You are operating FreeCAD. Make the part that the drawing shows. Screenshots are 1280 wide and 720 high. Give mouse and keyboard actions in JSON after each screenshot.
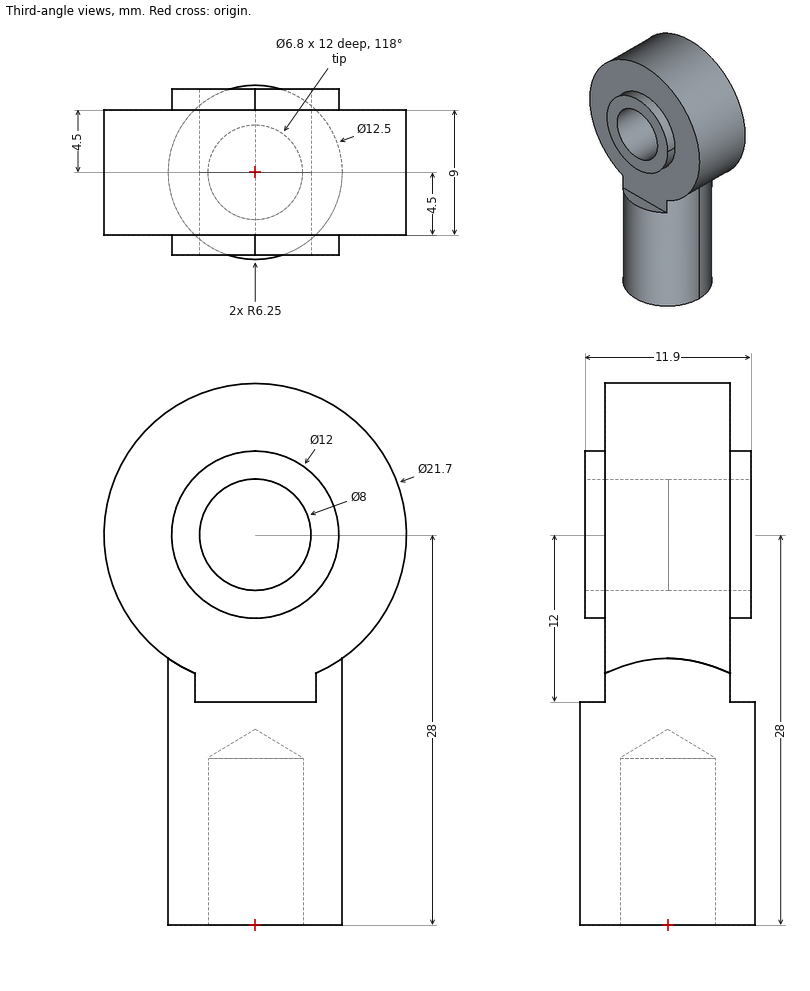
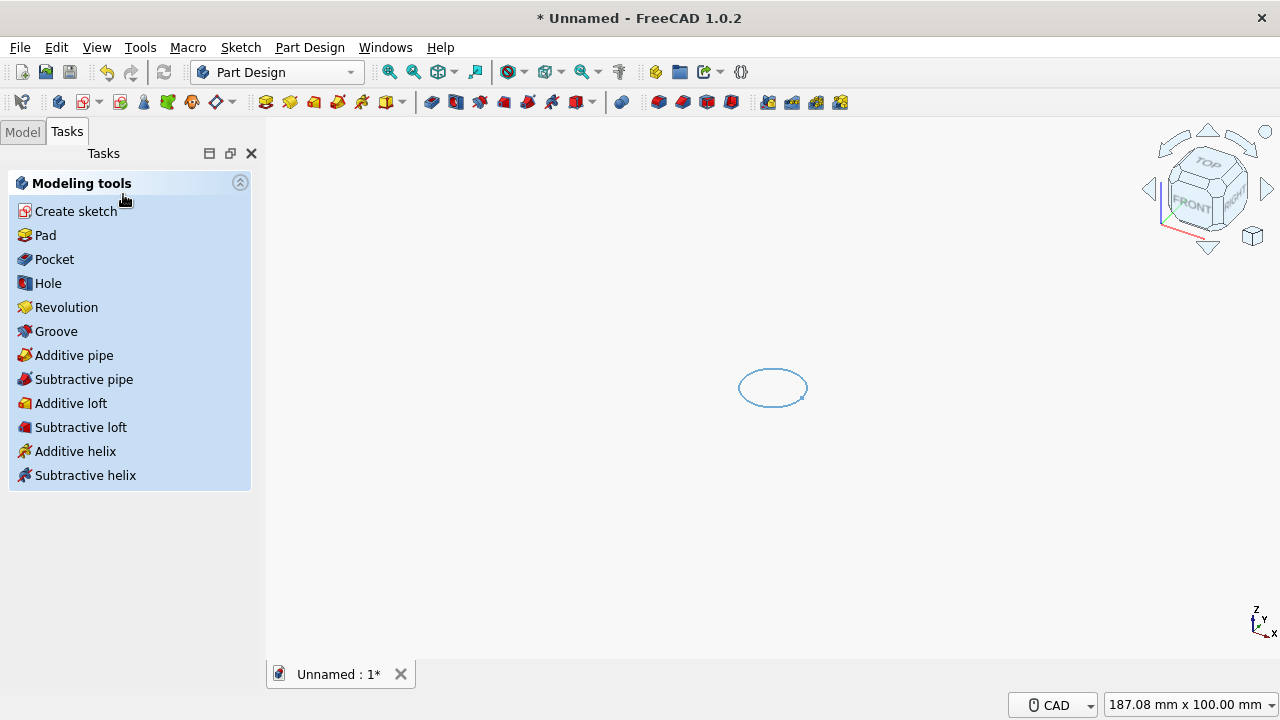
{"action": "left_click", "coordinate": [266, 102]}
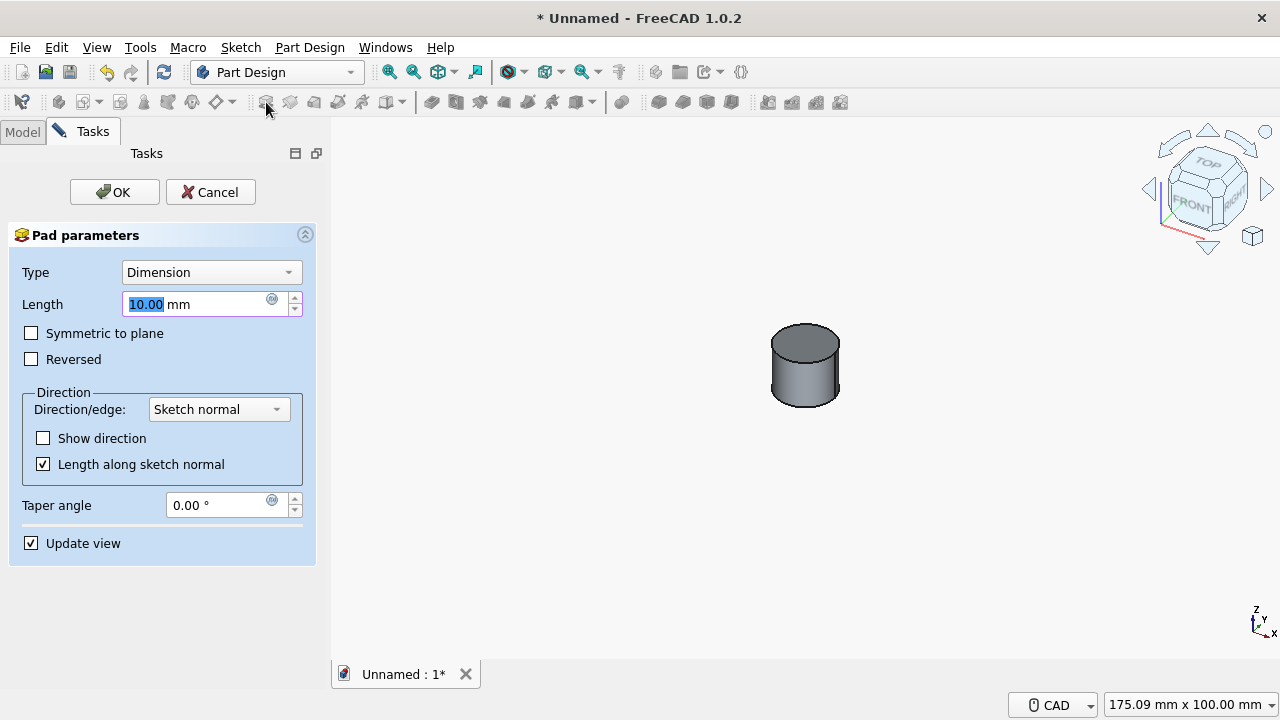
{"action": "type", "text": "28"}
{"action": "key", "text": "Tab"}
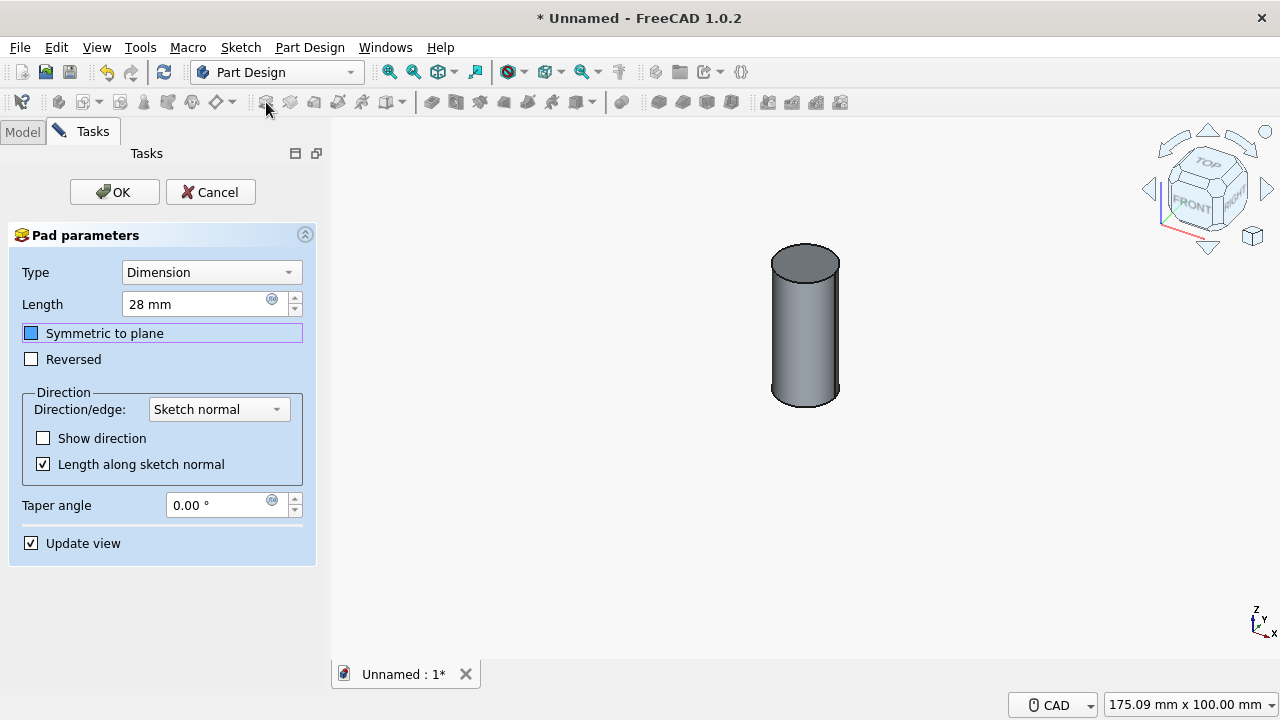
{"action": "left_click", "coordinate": [115, 192]}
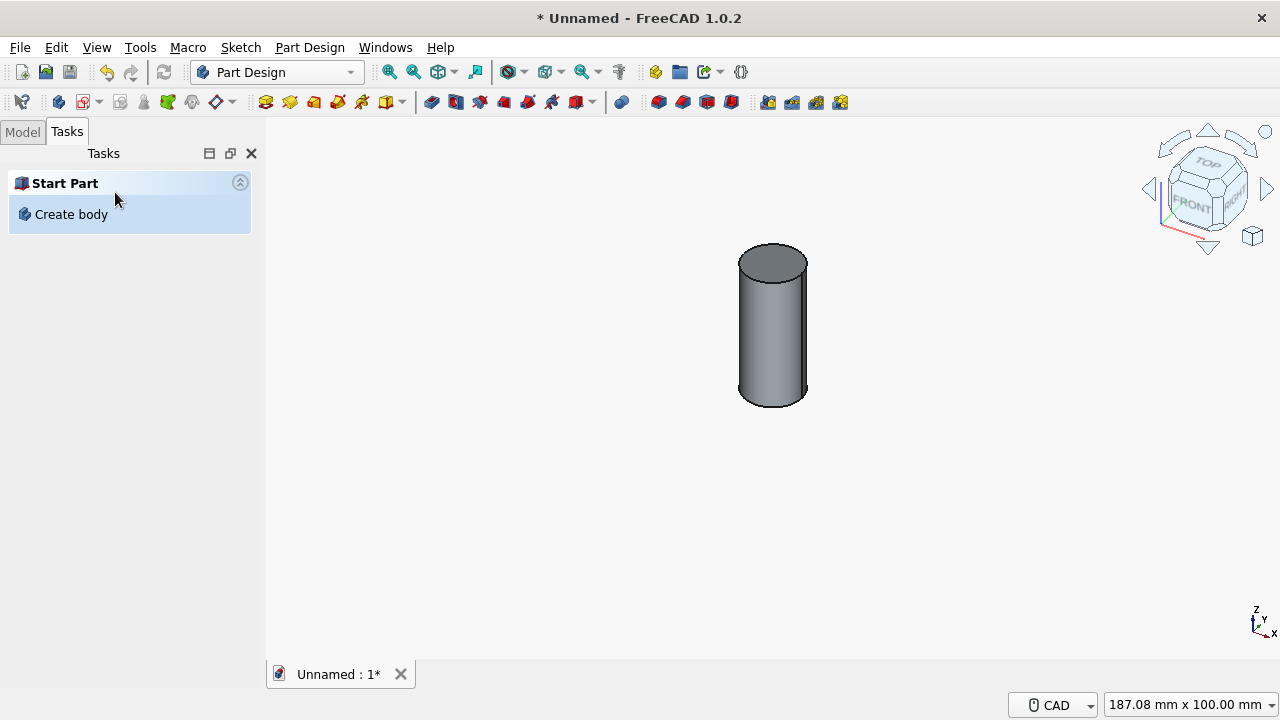
{"action": "left_click", "coordinate": [390, 72]}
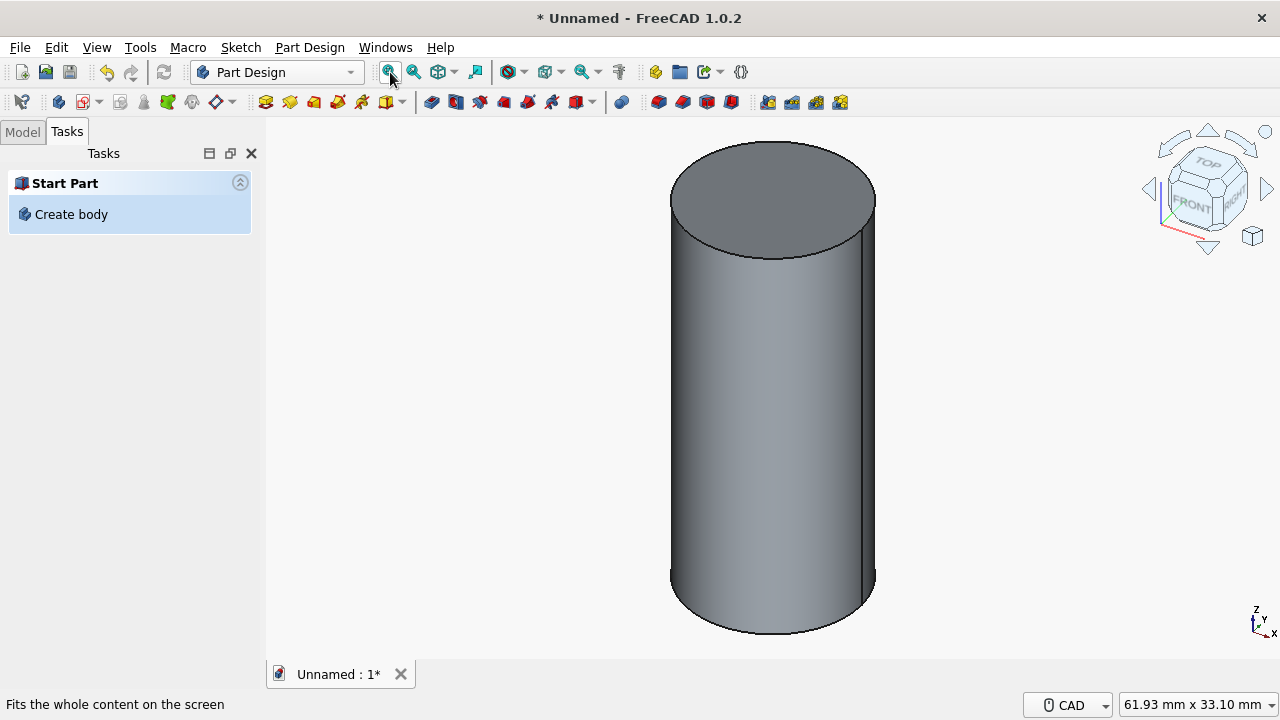
{"action": "left_click", "coordinate": [84, 102]}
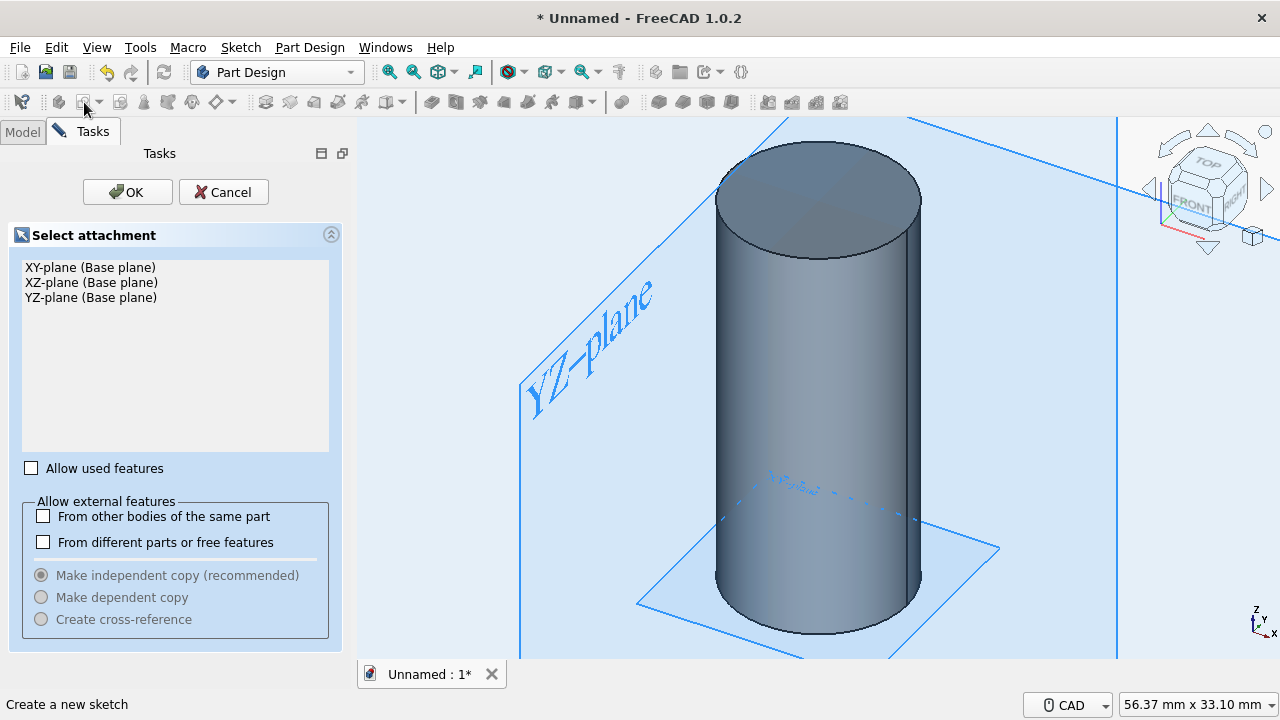
{"action": "left_click", "coordinate": [82, 282]}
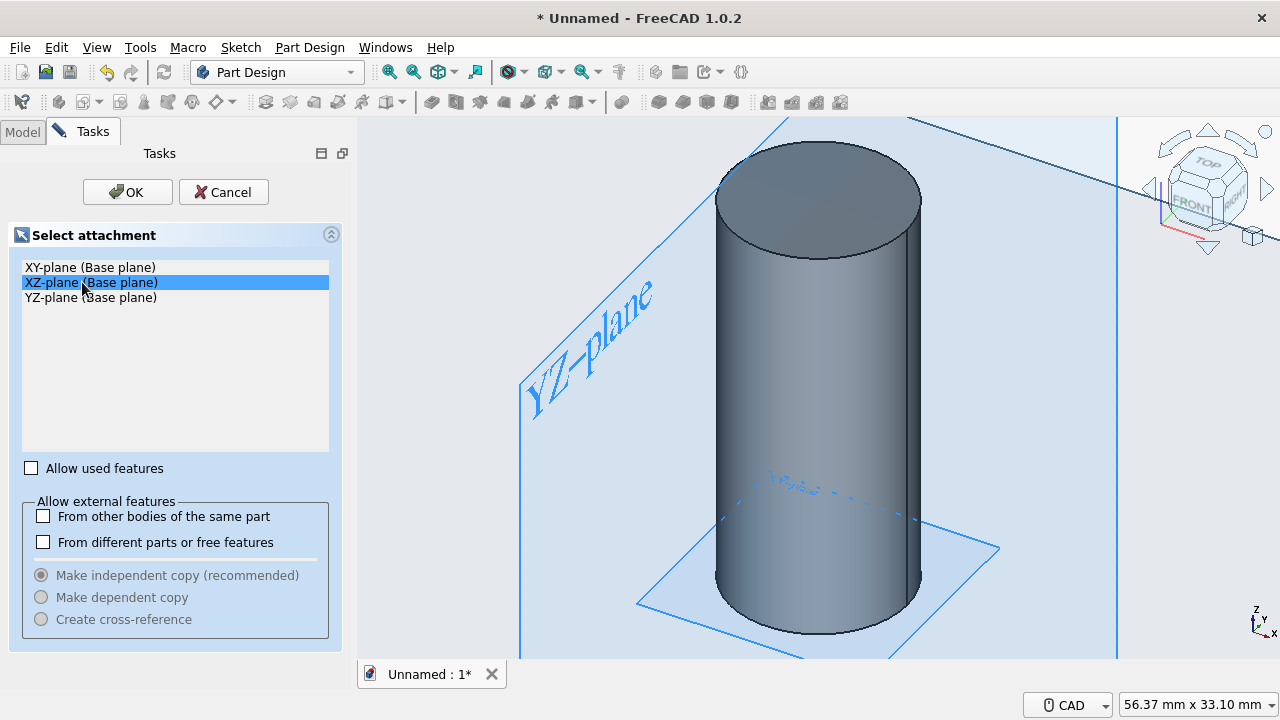
{"action": "left_click", "coordinate": [128, 192]}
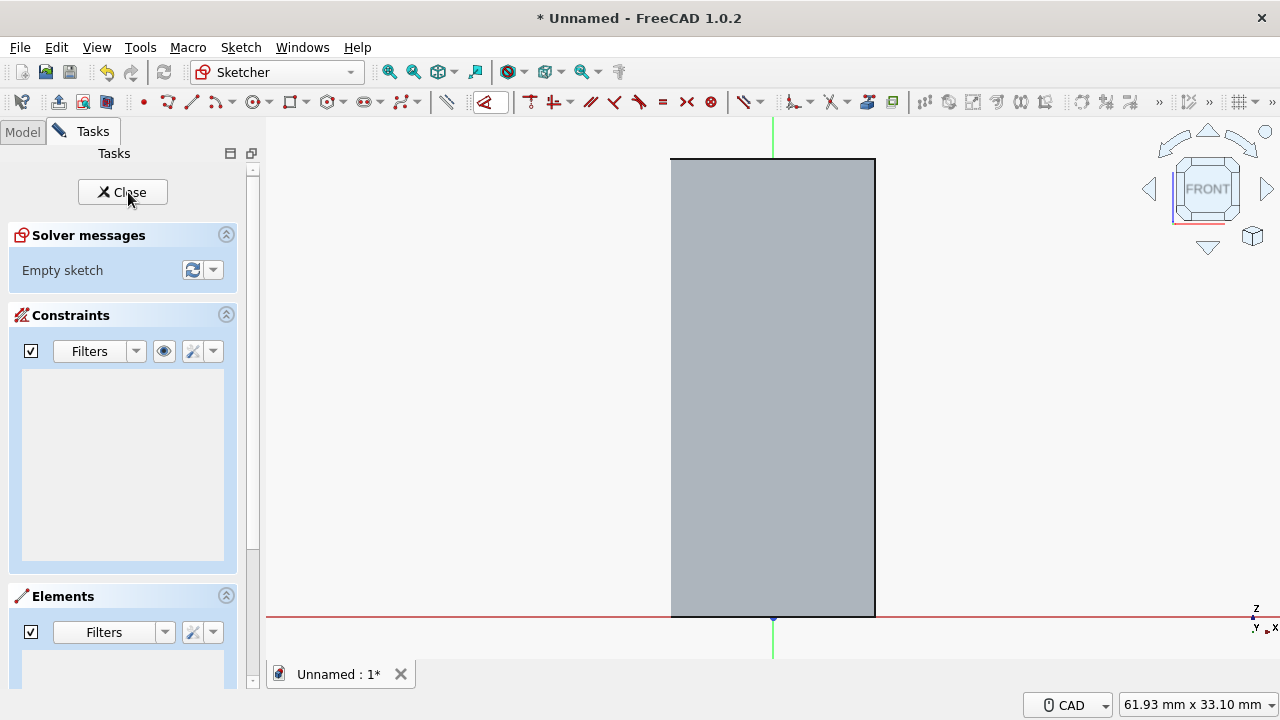
{"action": "left_click", "coordinate": [108, 102]}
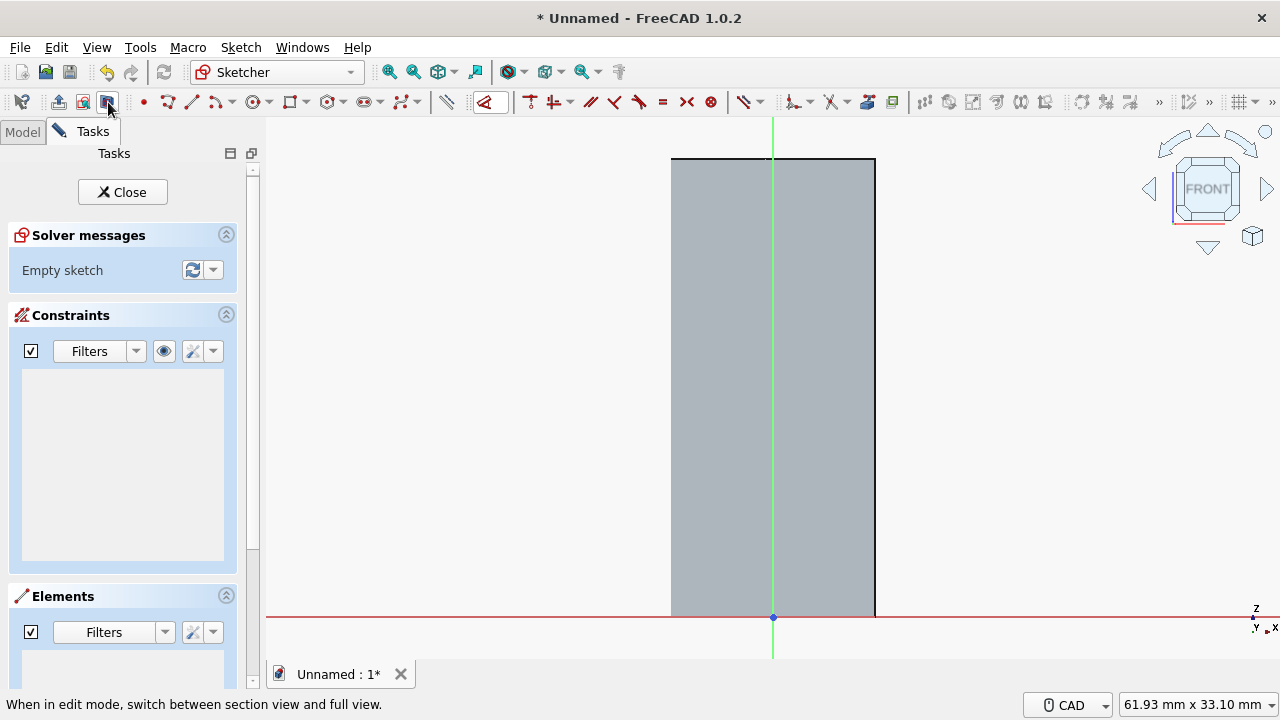
{"action": "scroll", "coordinate": [621, 496], "scroll_direction": "down", "scroll_amount": 3}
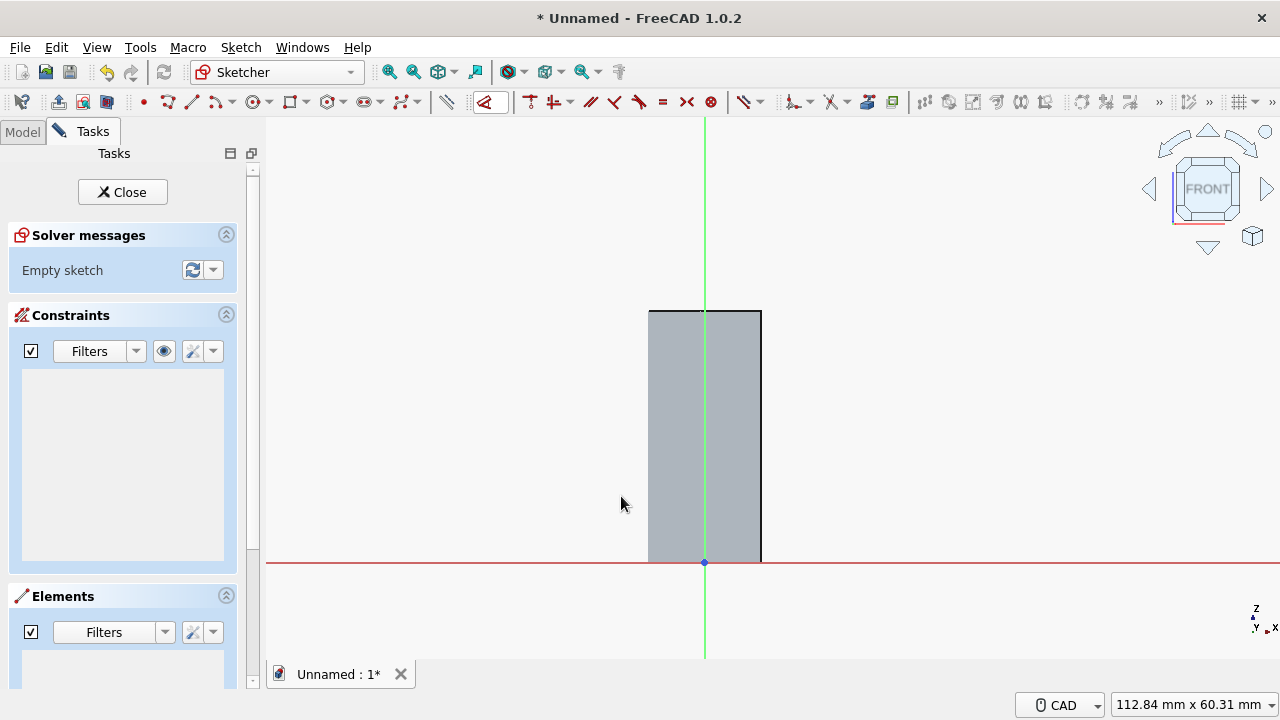
{"action": "left_click", "coordinate": [254, 102]}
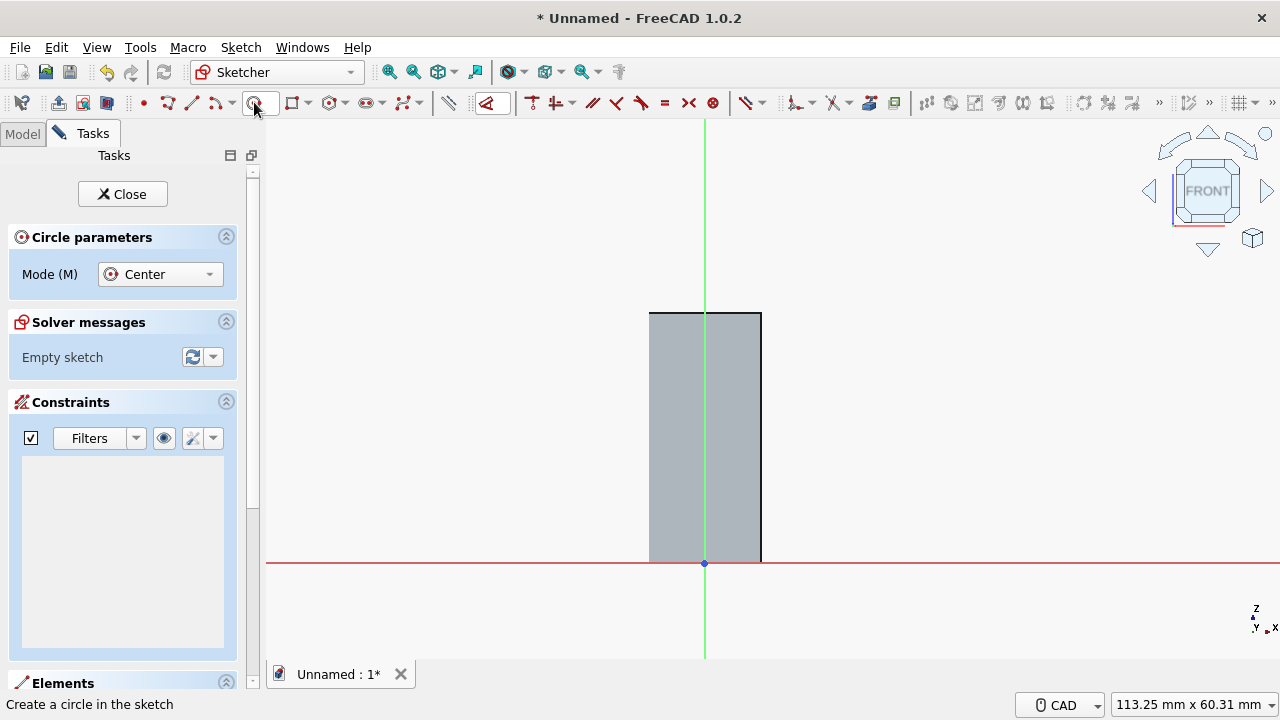
{"action": "left_click", "coordinate": [705, 313]}
{"action": "left_click", "coordinate": [774, 244]}
{"action": "key", "text": "Escape"}